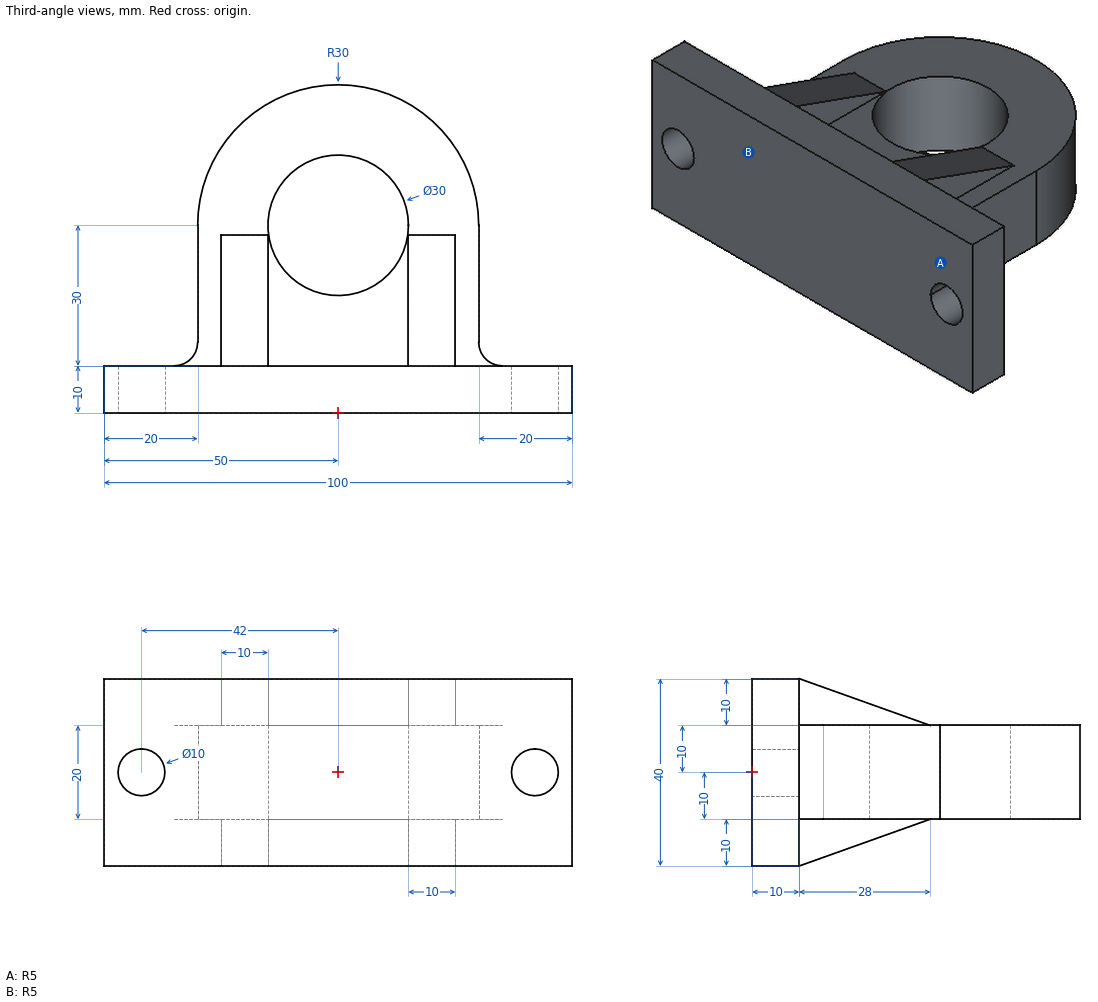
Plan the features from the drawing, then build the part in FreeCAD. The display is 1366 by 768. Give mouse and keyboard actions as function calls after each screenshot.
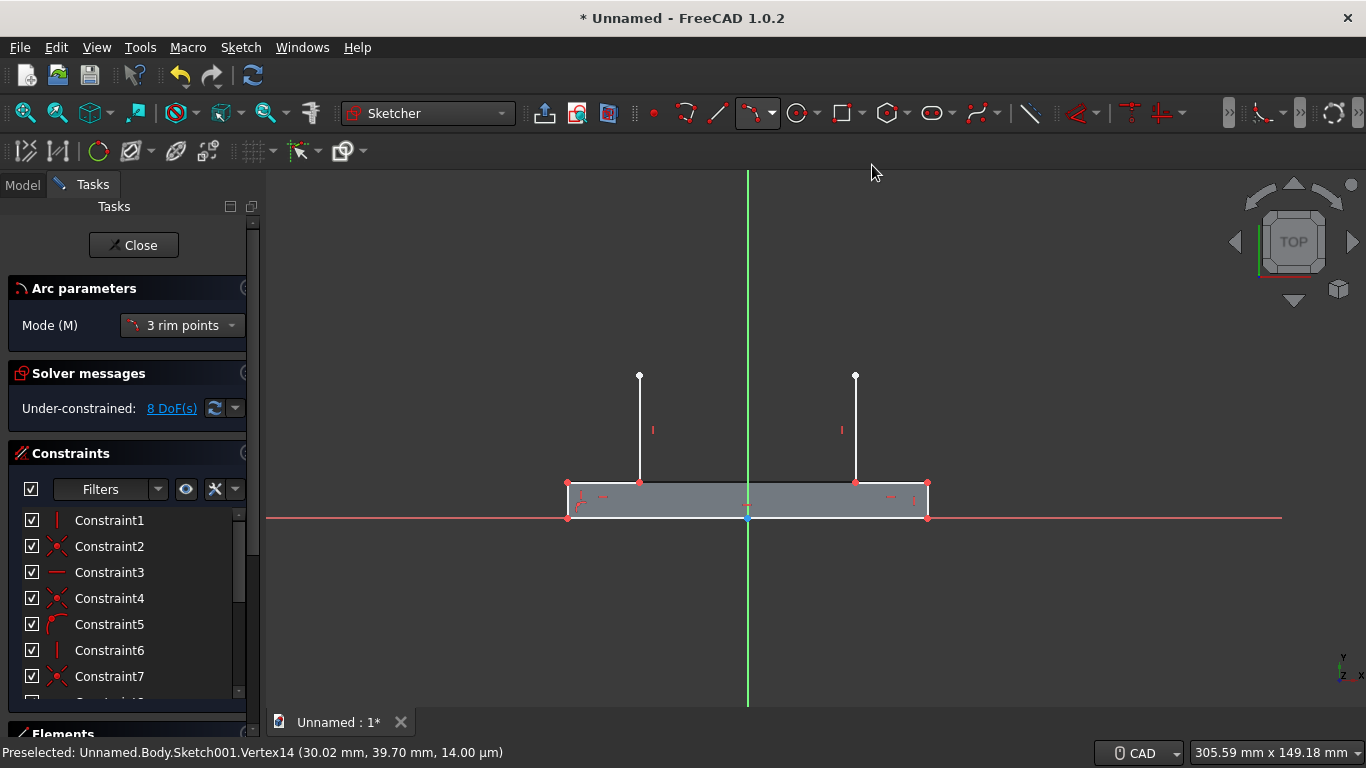
click(856, 375)
click(640, 375)
click(781, 271)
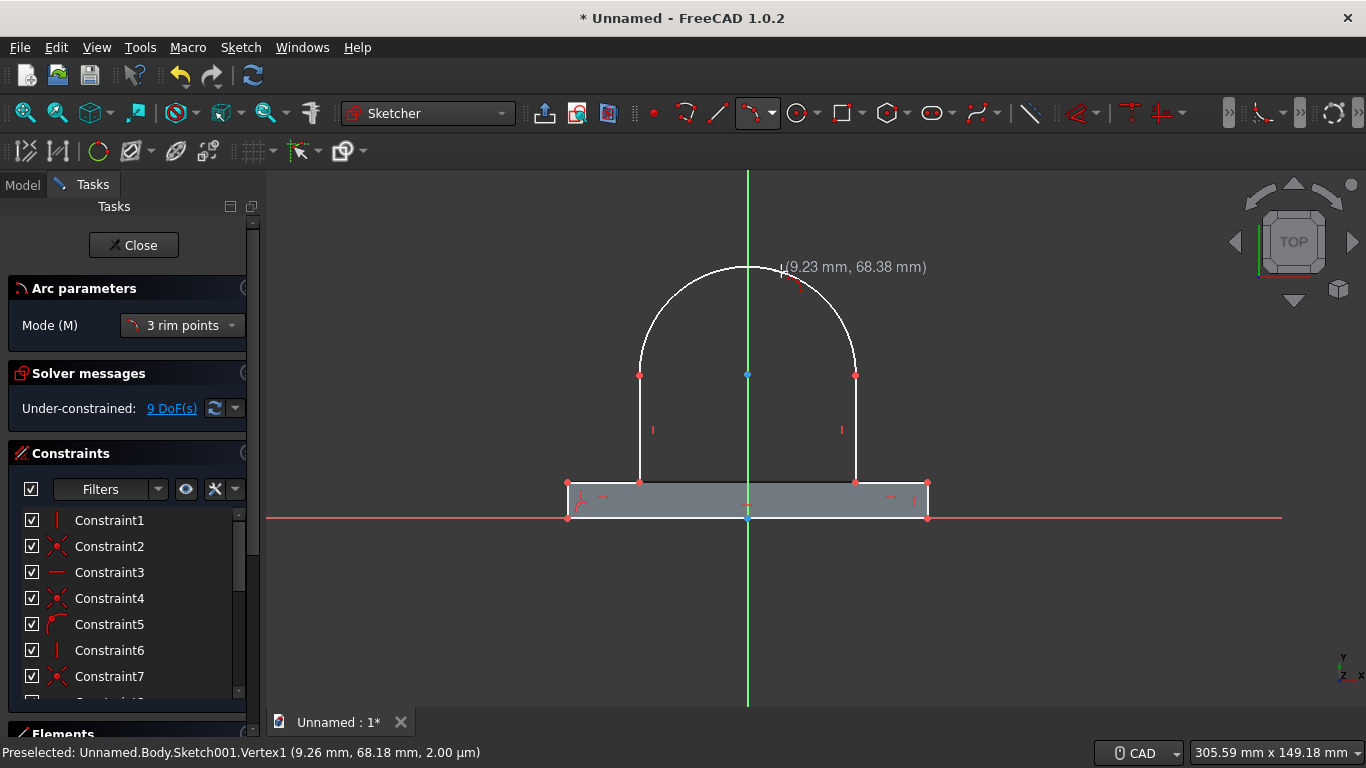
click(798, 114)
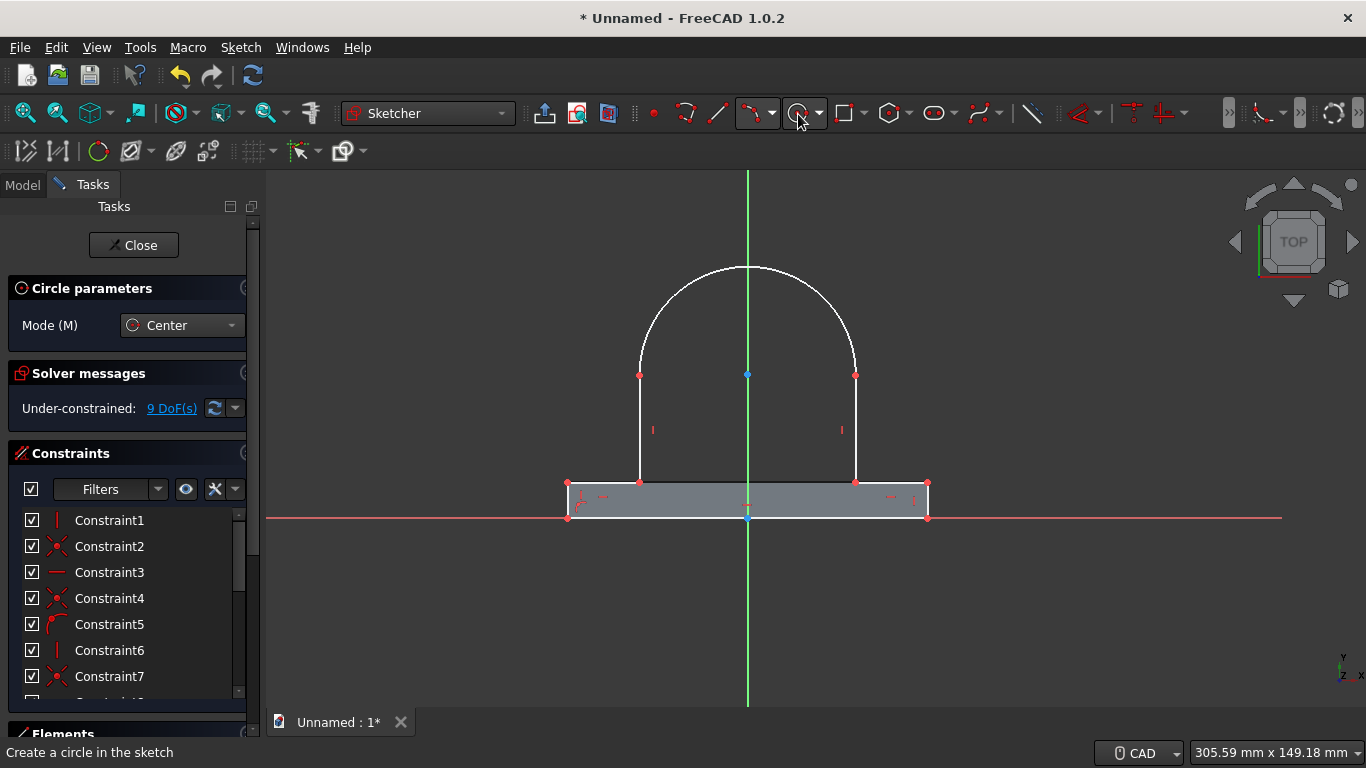
click(748, 374)
move(786, 336)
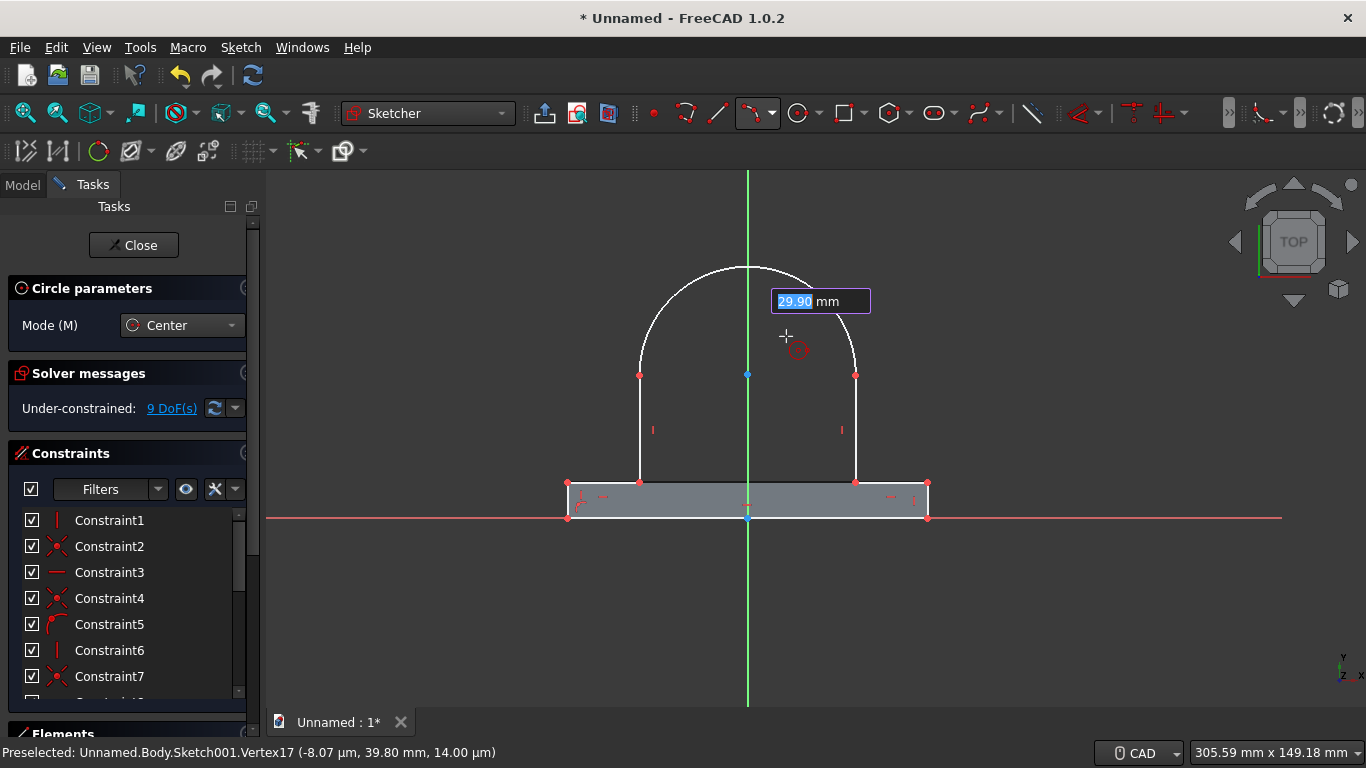
text(30)
key(Return)
key(Escape)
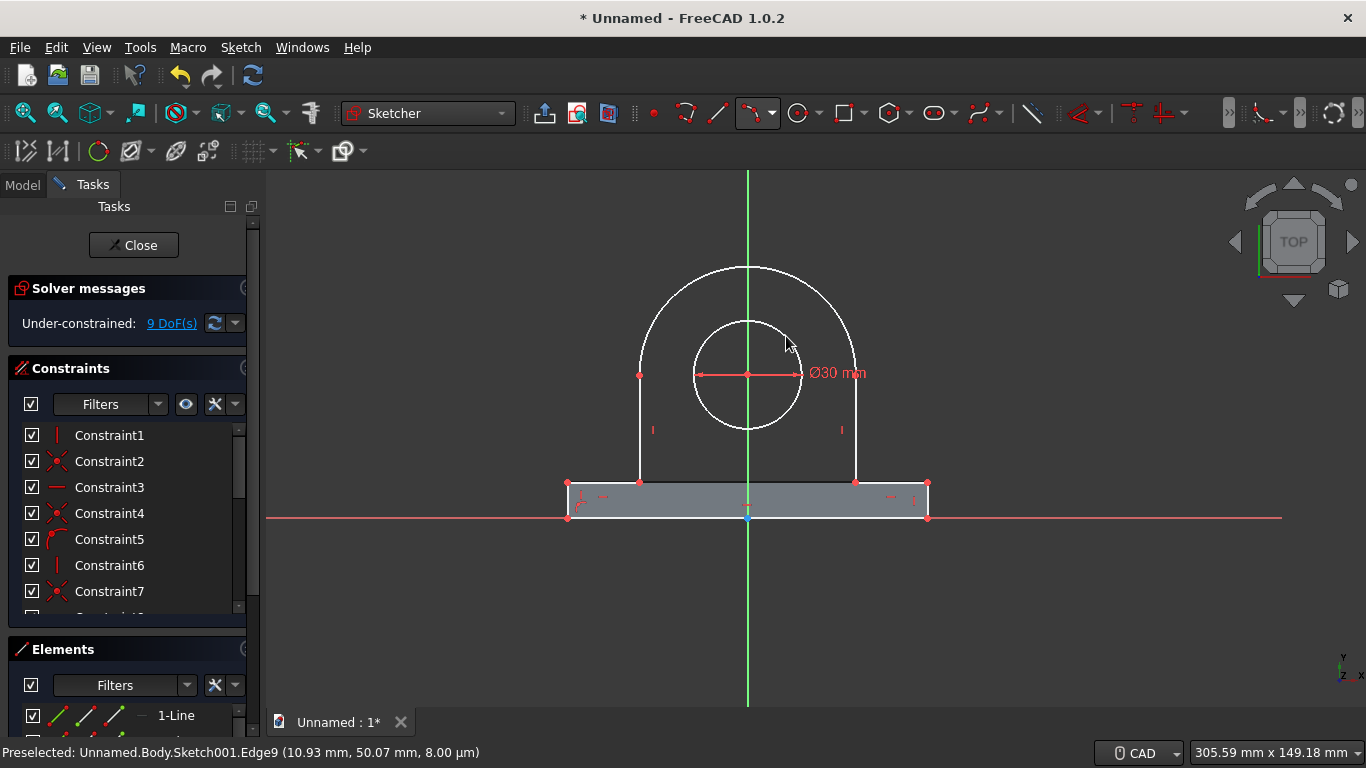
click(640, 408)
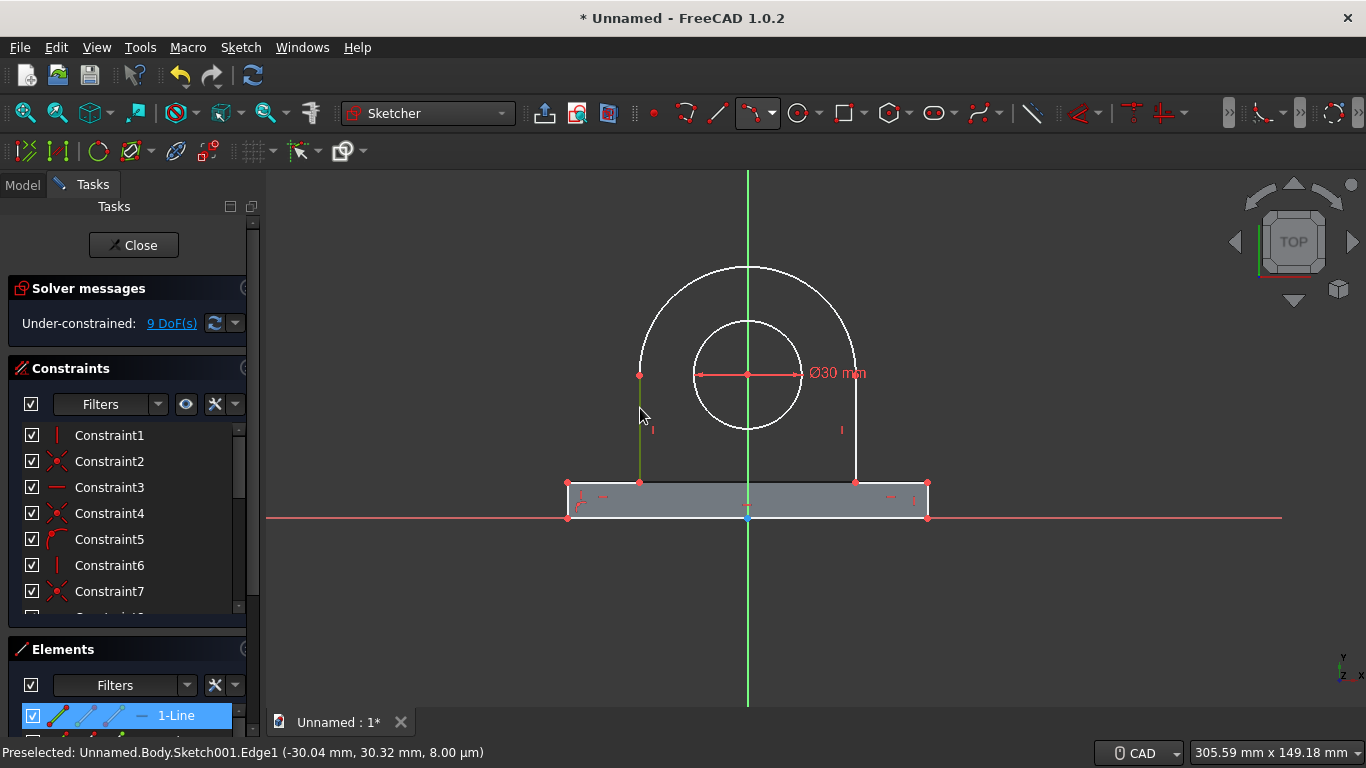
click(811, 287)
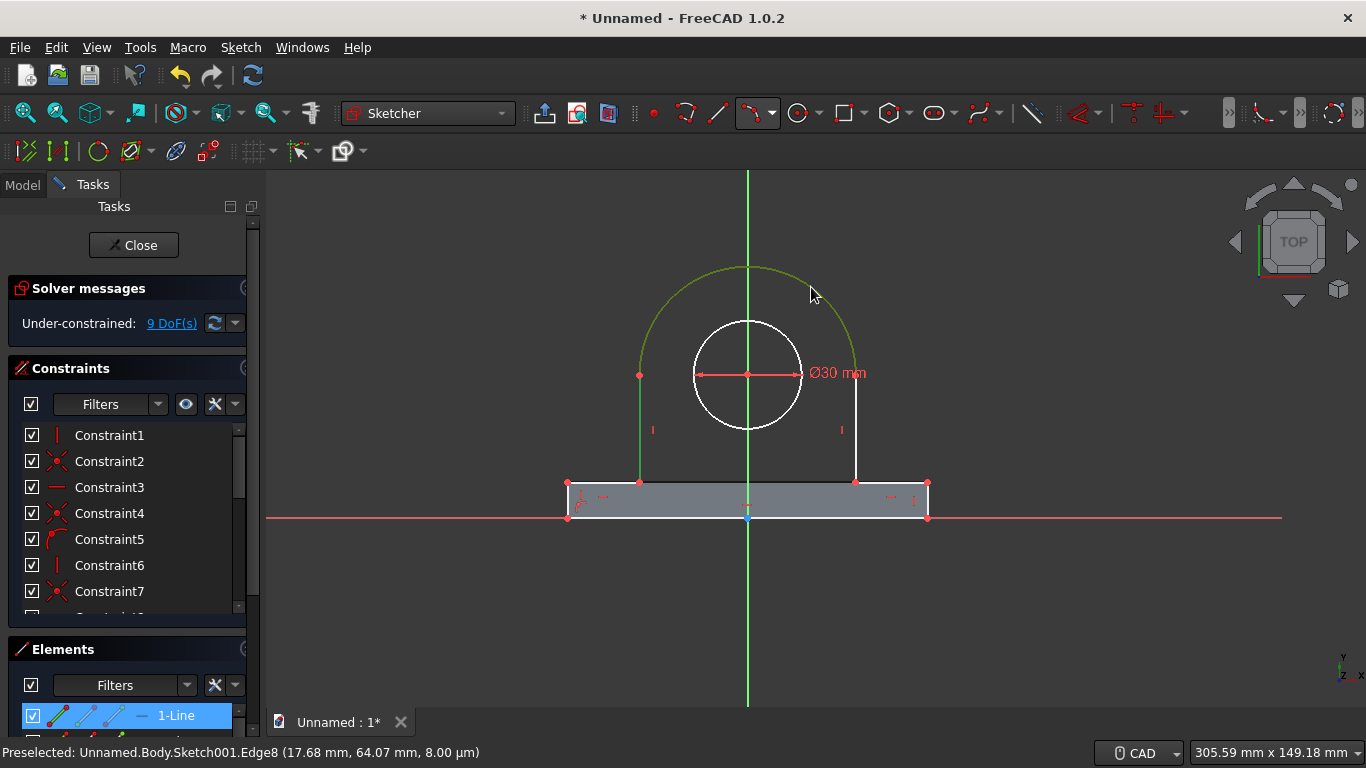
key(t)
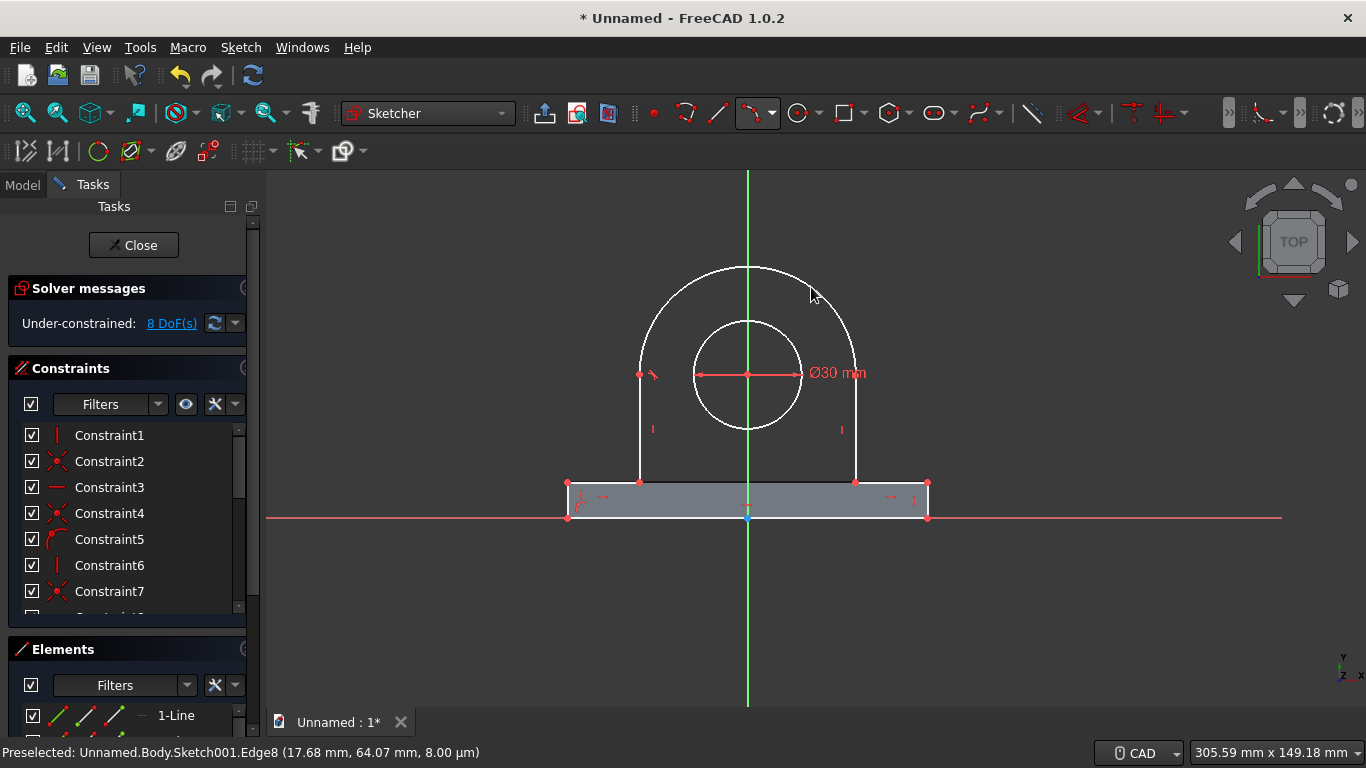
click(856, 451)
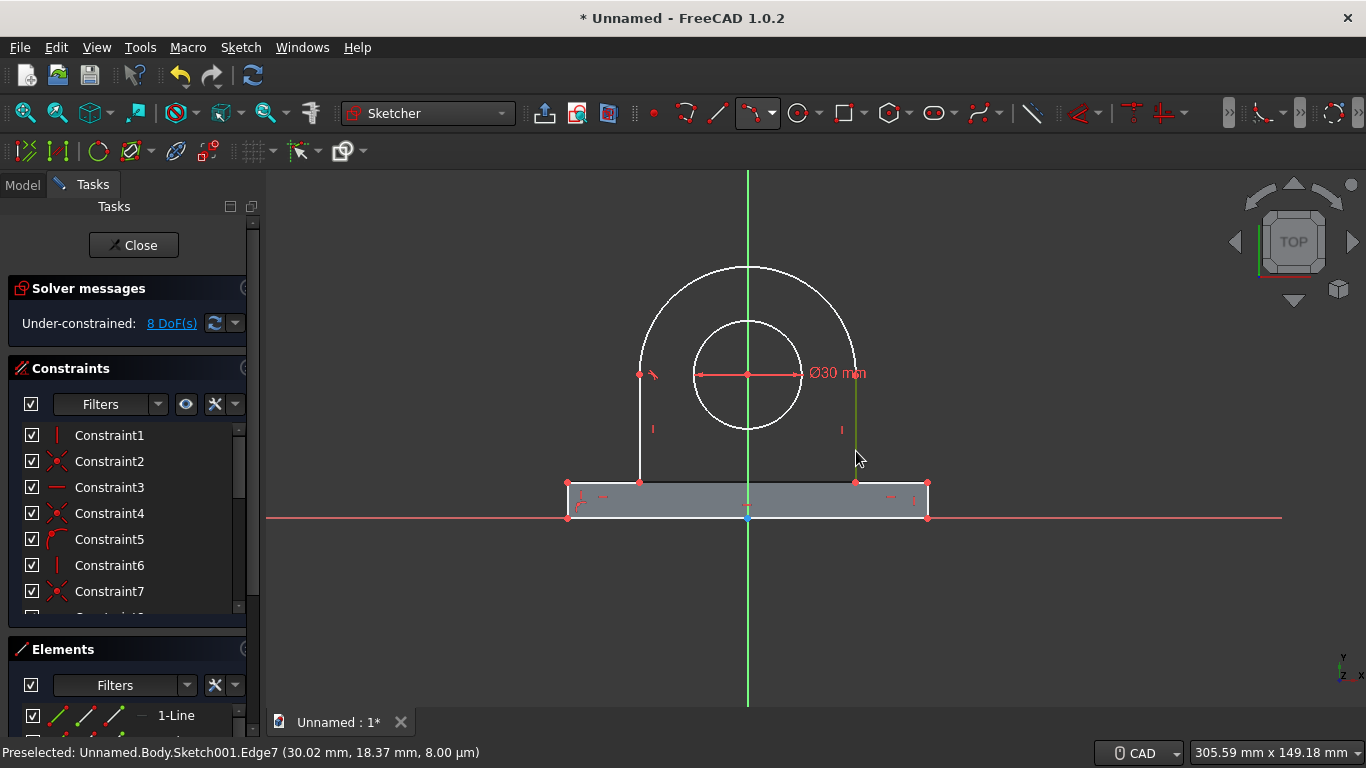
click(812, 288)